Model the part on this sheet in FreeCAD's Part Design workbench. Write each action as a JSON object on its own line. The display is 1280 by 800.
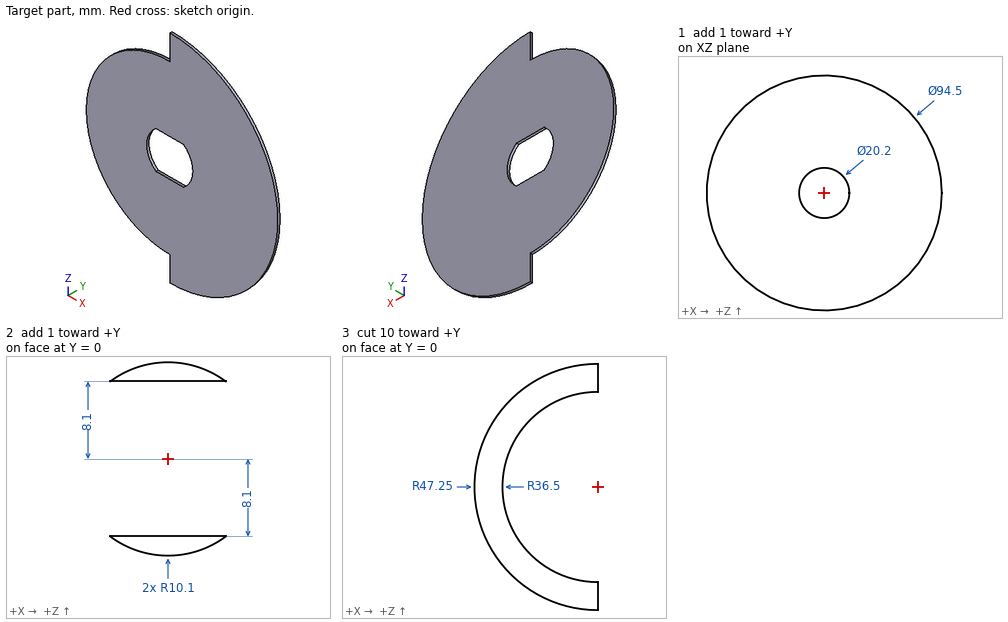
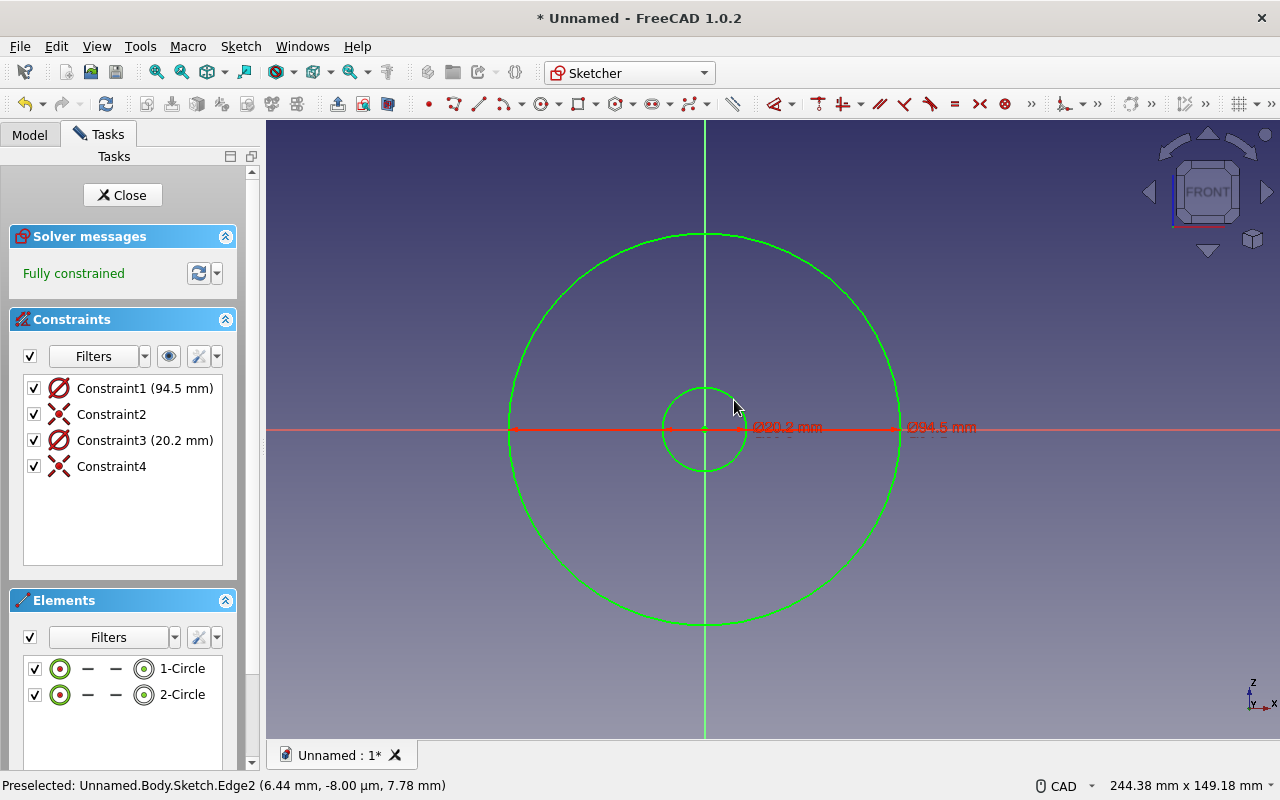
{"action": "left_click", "coordinate": [123, 195]}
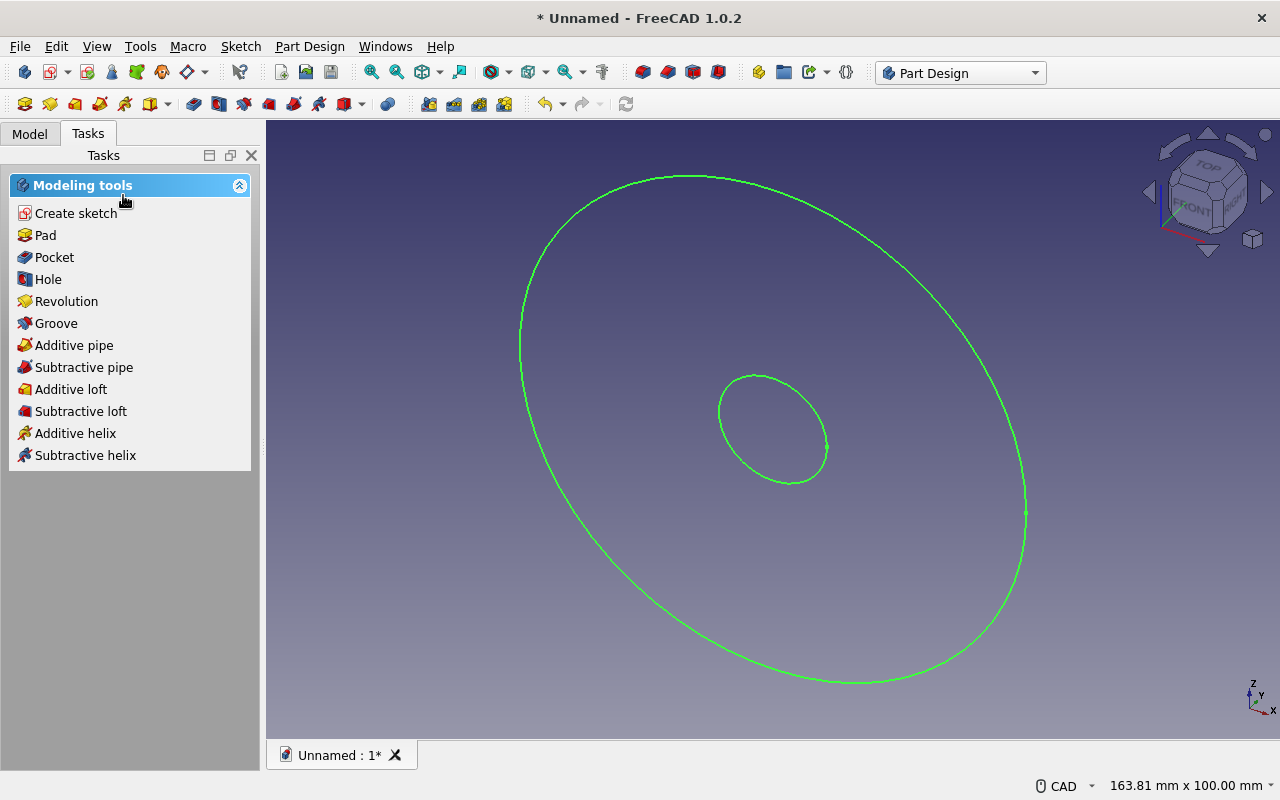
{"action": "left_click", "coordinate": [25, 104]}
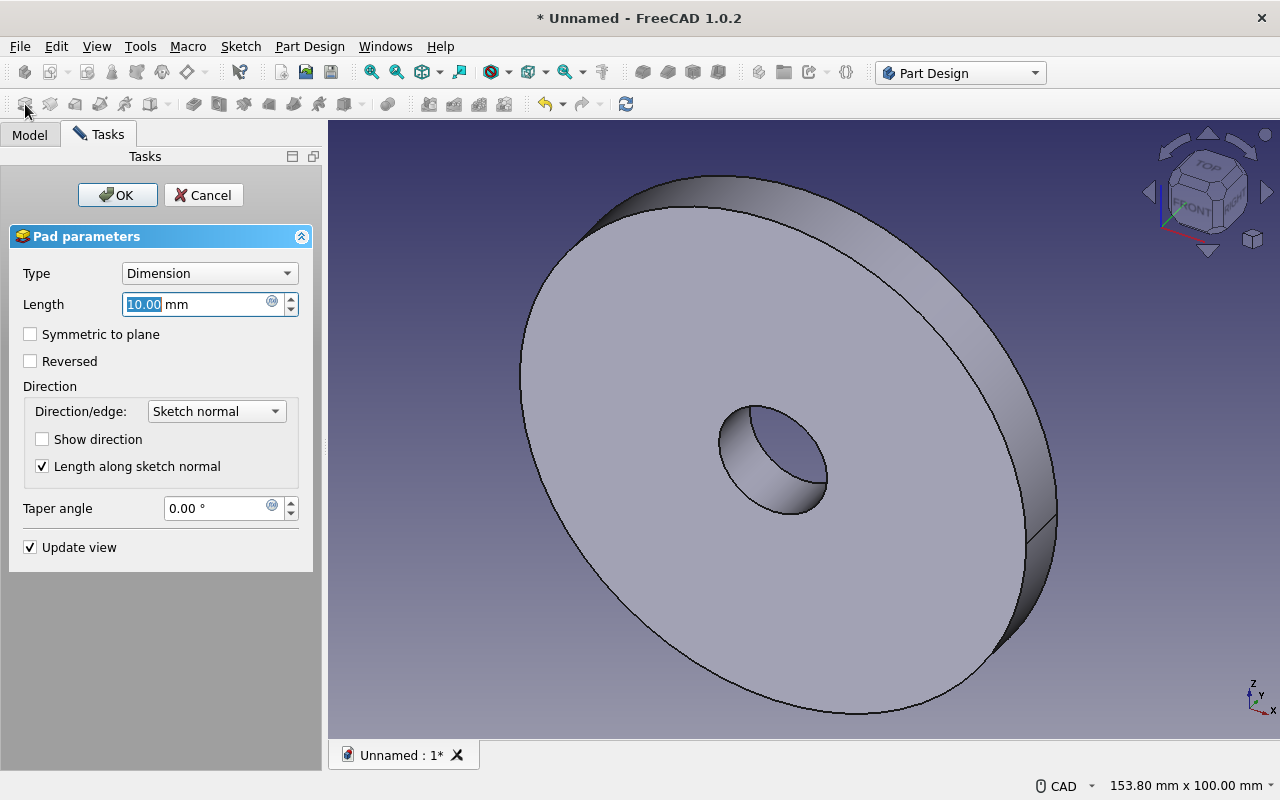
{"action": "type", "text": "1"}
{"action": "key", "text": "Tab"}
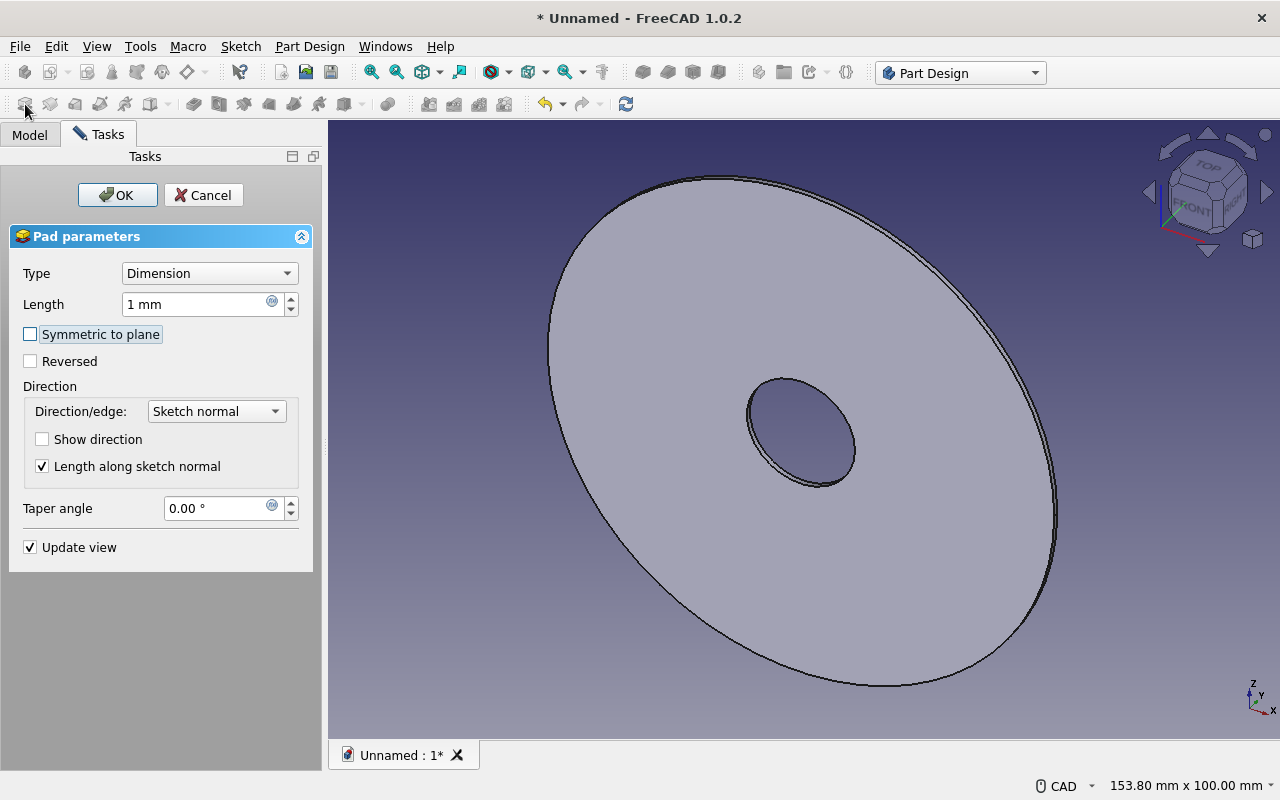
{"action": "left_click", "coordinate": [31, 361]}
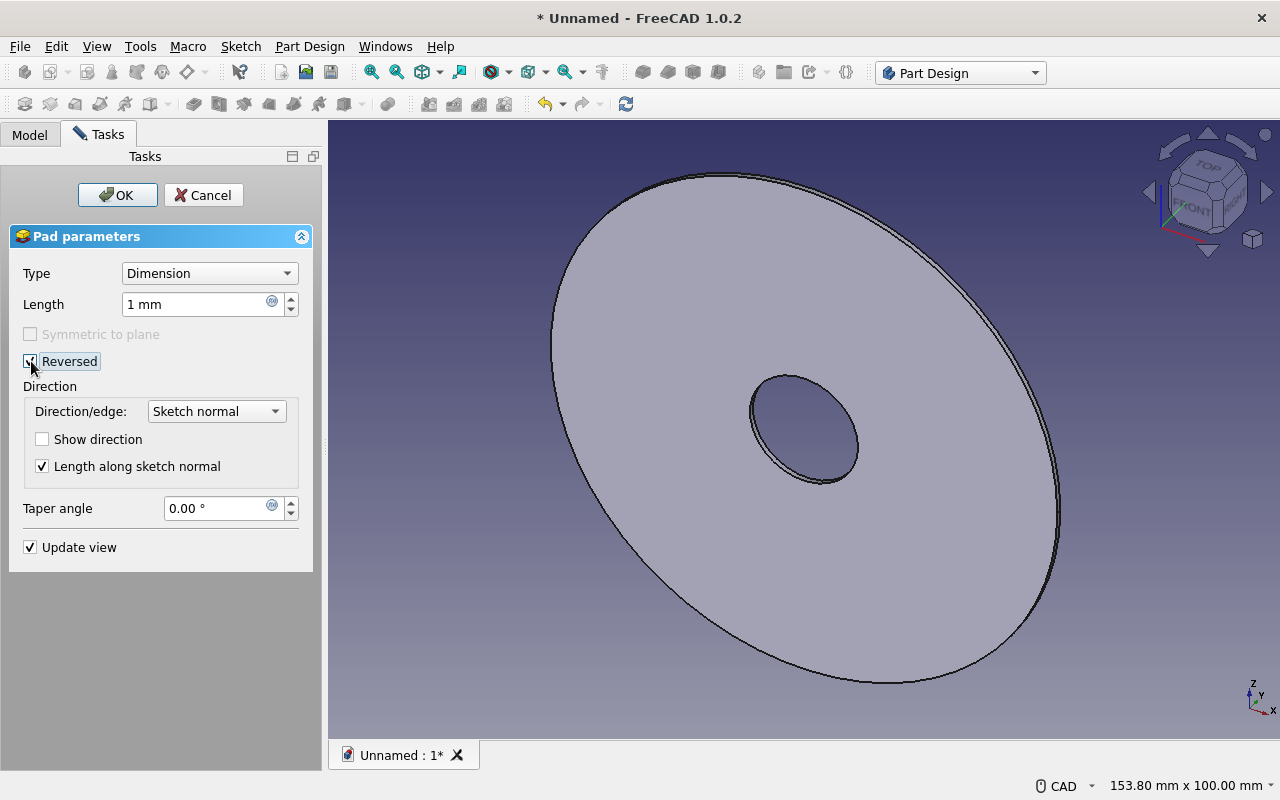
{"action": "left_click", "coordinate": [118, 195]}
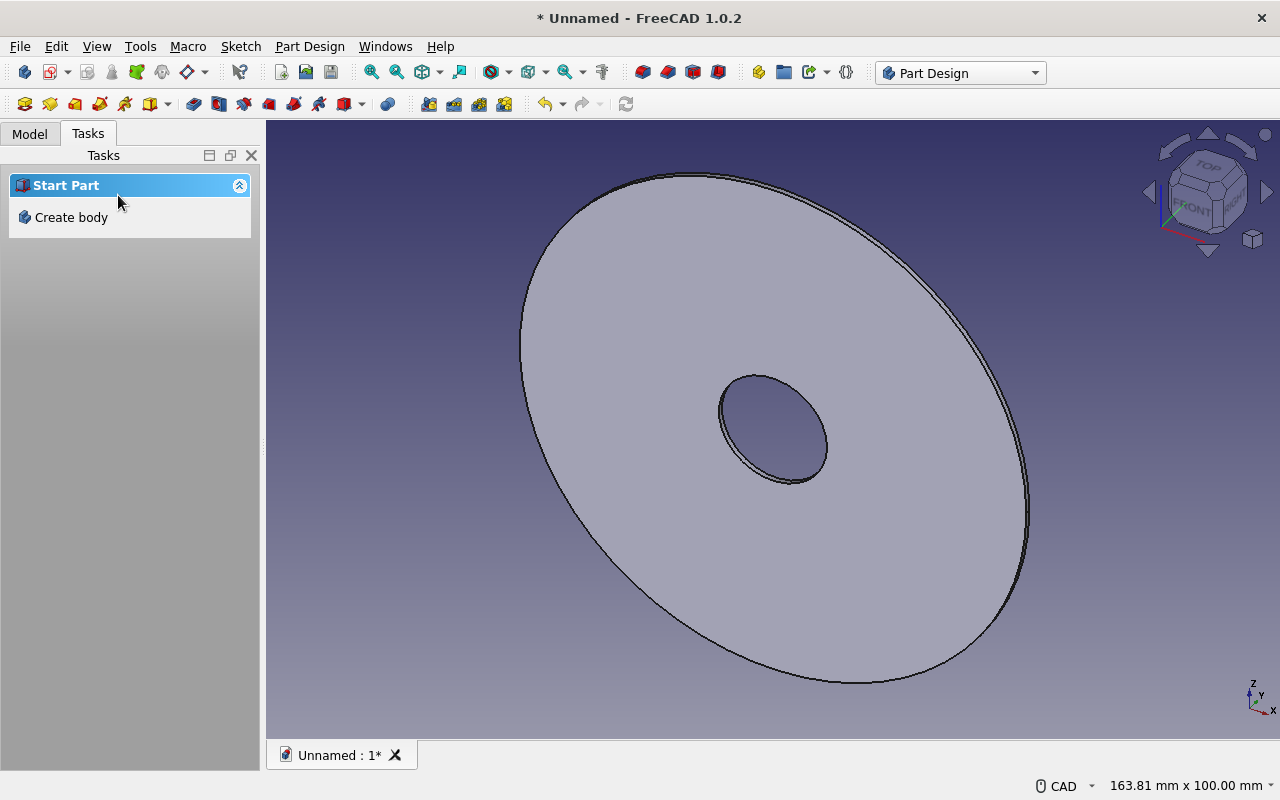
{"action": "left_click", "coordinate": [372, 72]}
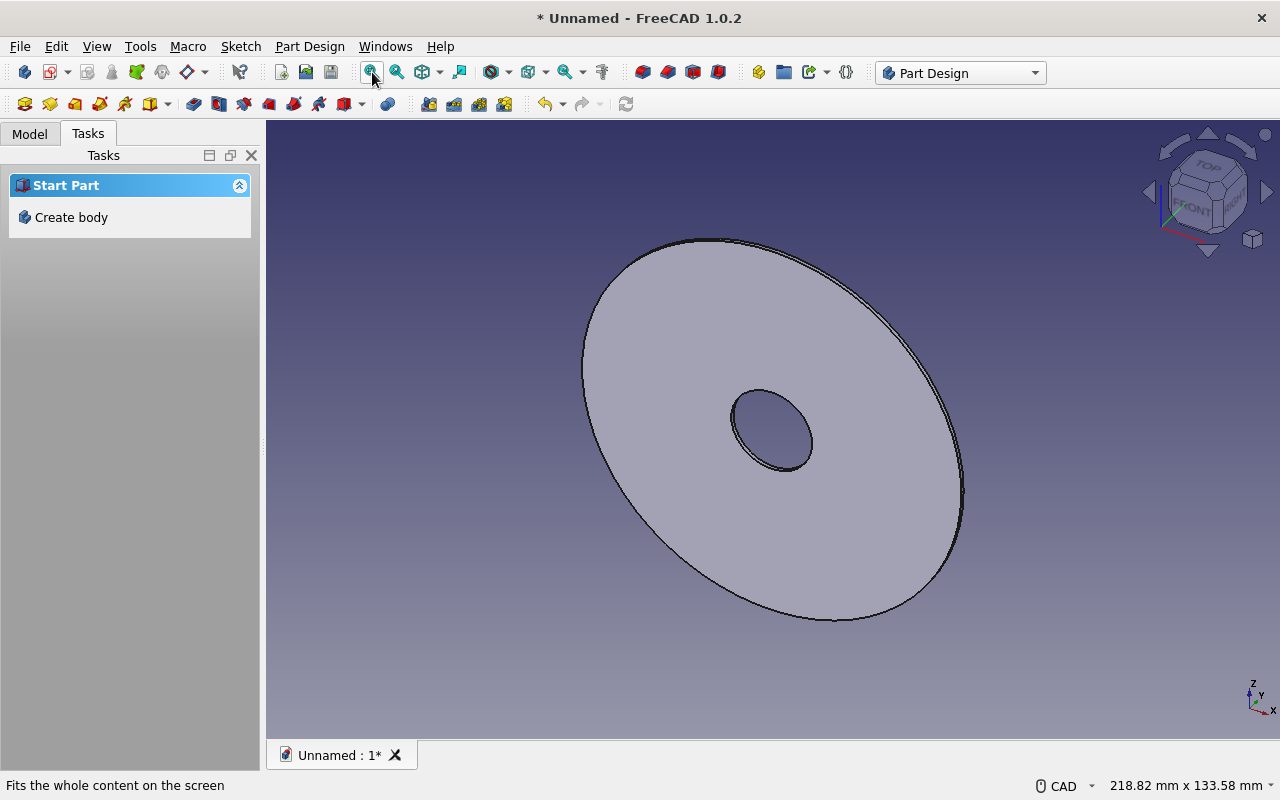
{"action": "left_click", "coordinate": [826, 345]}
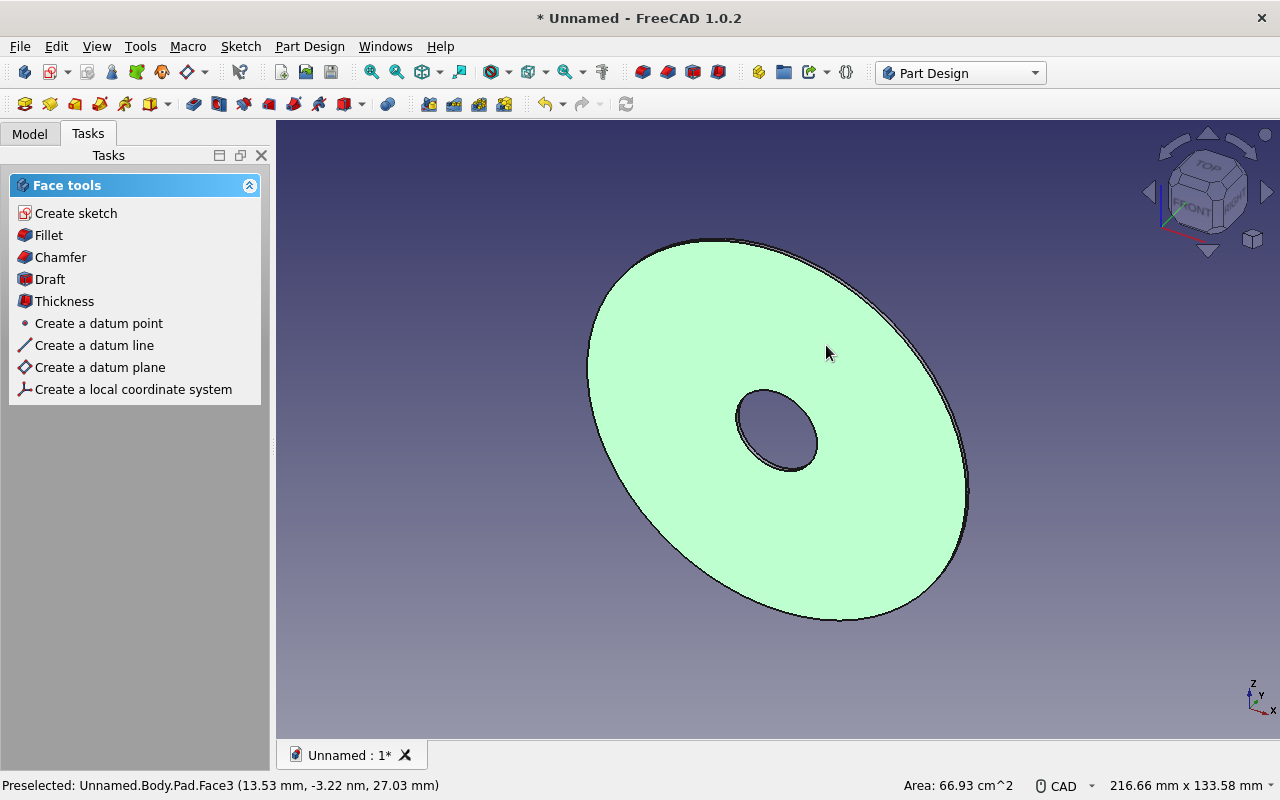
{"action": "left_click", "coordinate": [50, 72]}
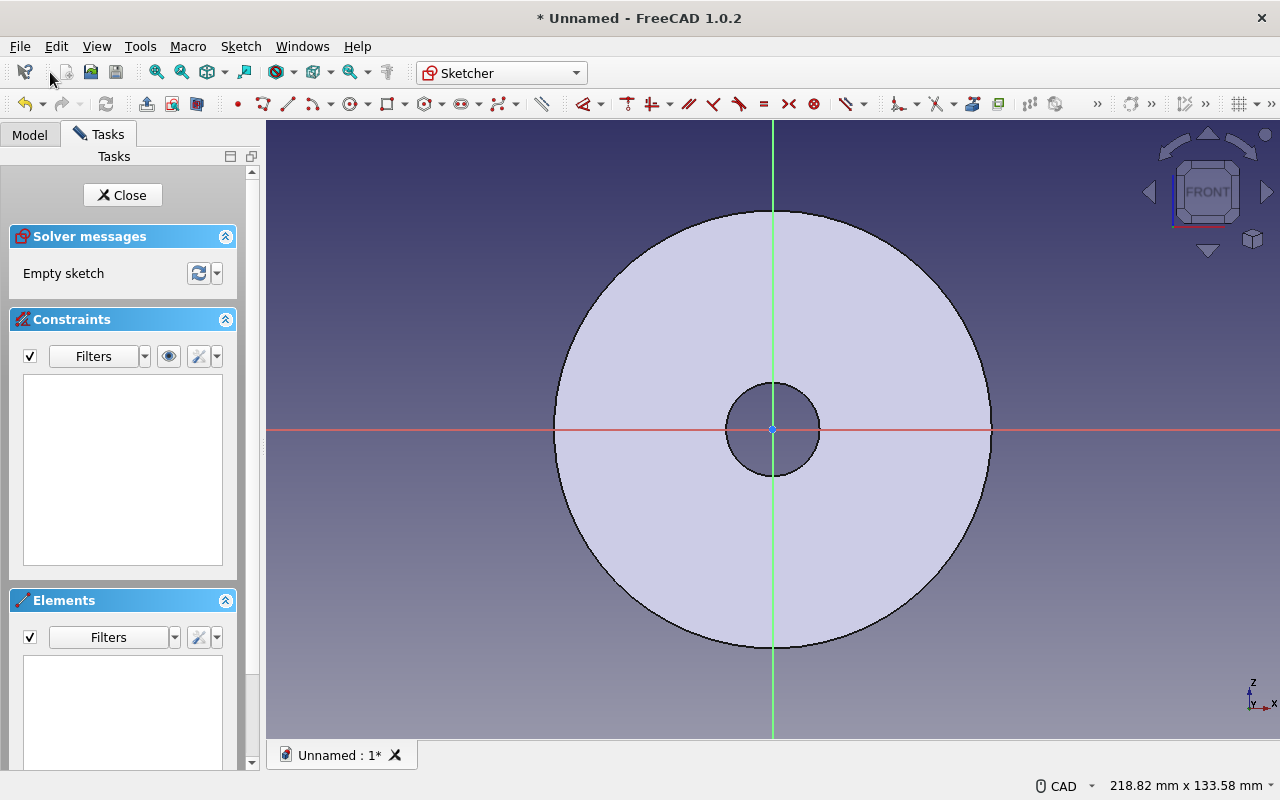
{"action": "scroll", "coordinate": [795, 430], "scroll_direction": "up", "scroll_amount": 7}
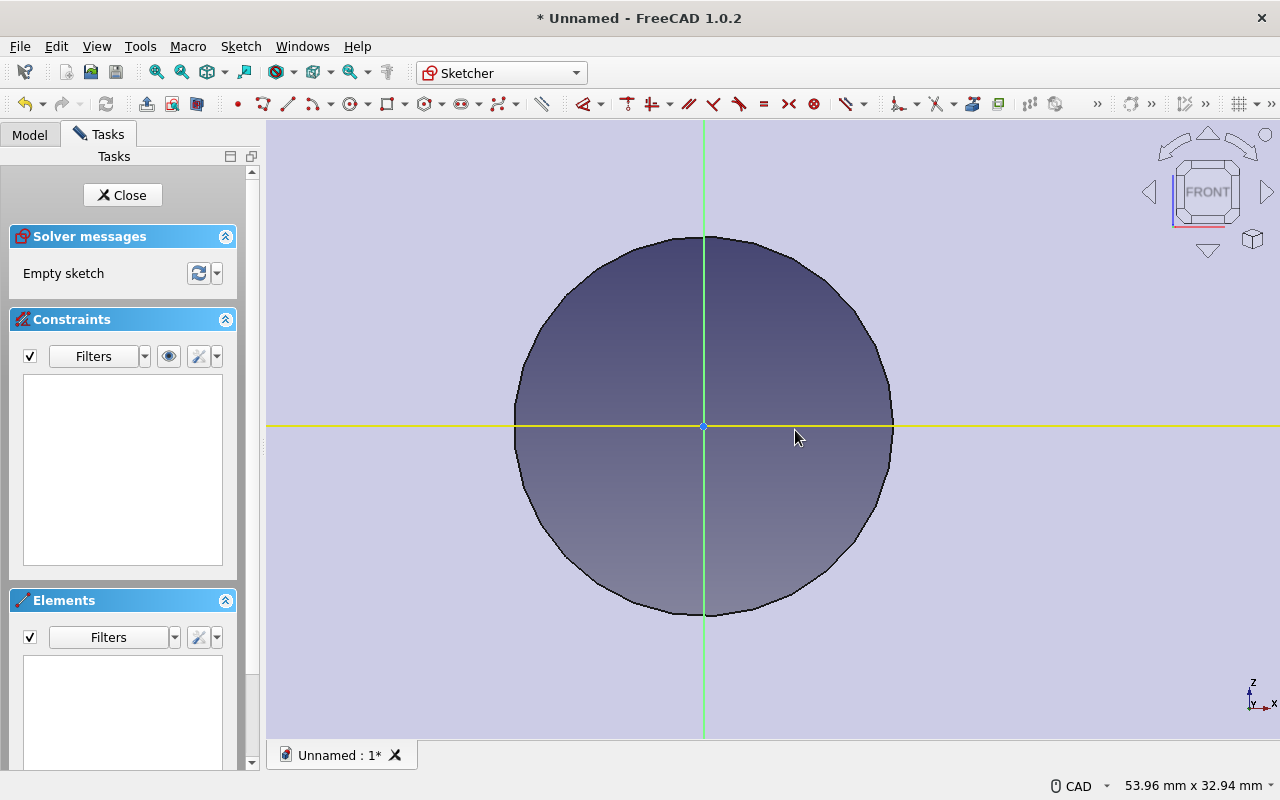
{"action": "left_click", "coordinate": [288, 104]}